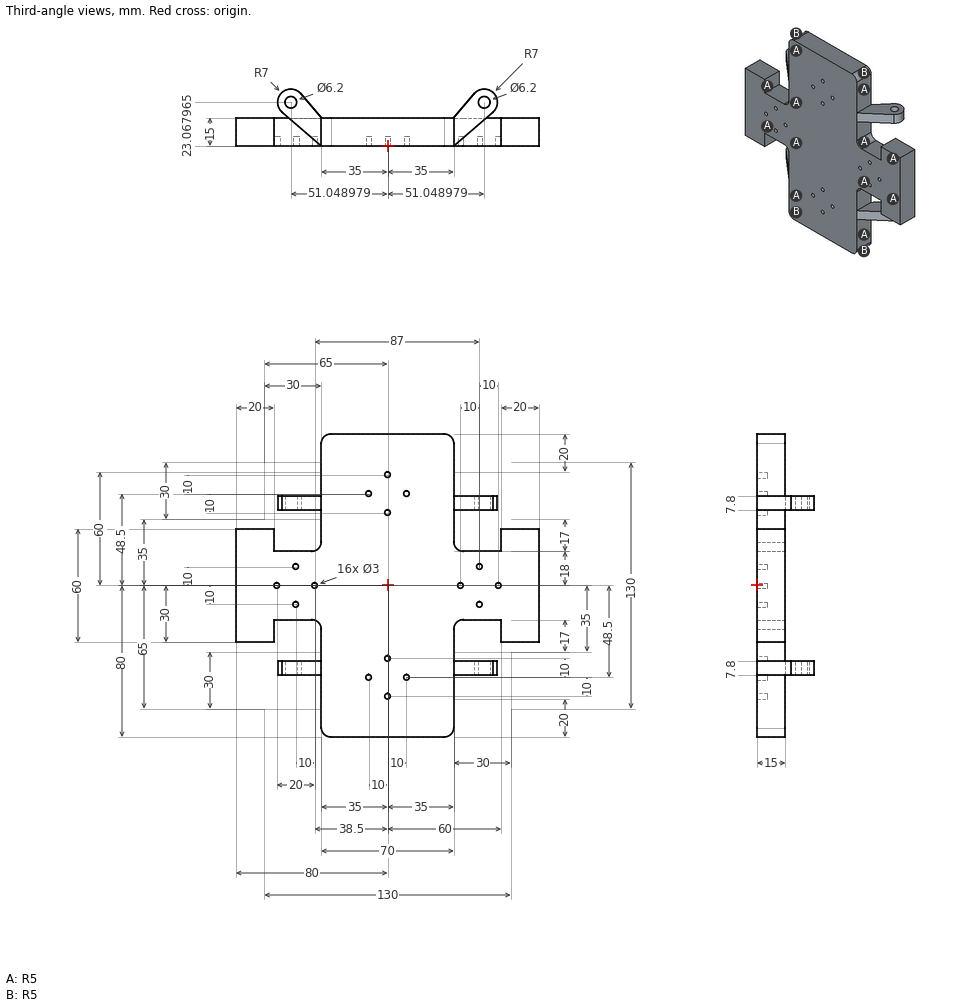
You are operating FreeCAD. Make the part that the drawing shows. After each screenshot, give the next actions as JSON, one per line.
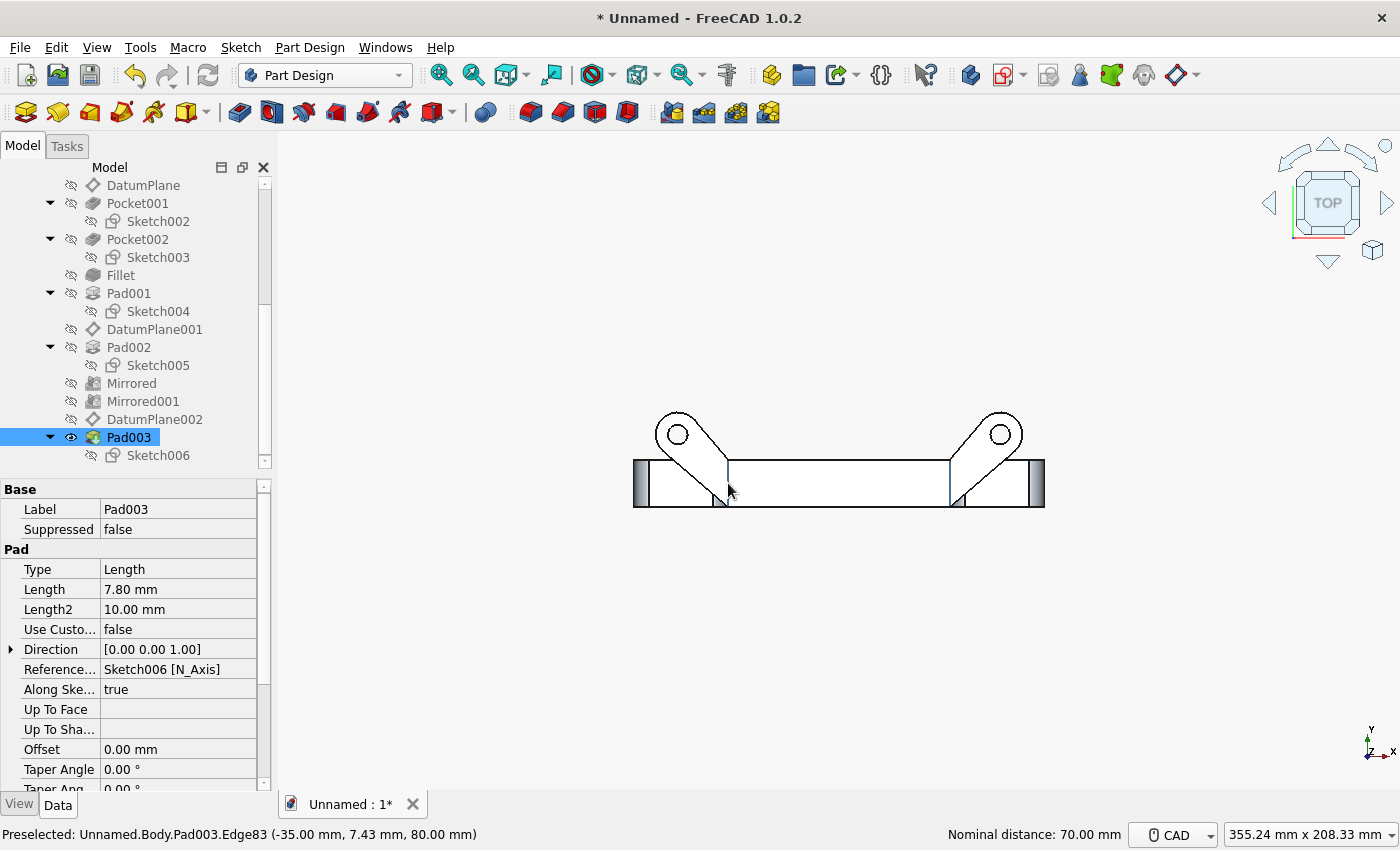
{"action": "key", "text": "1"}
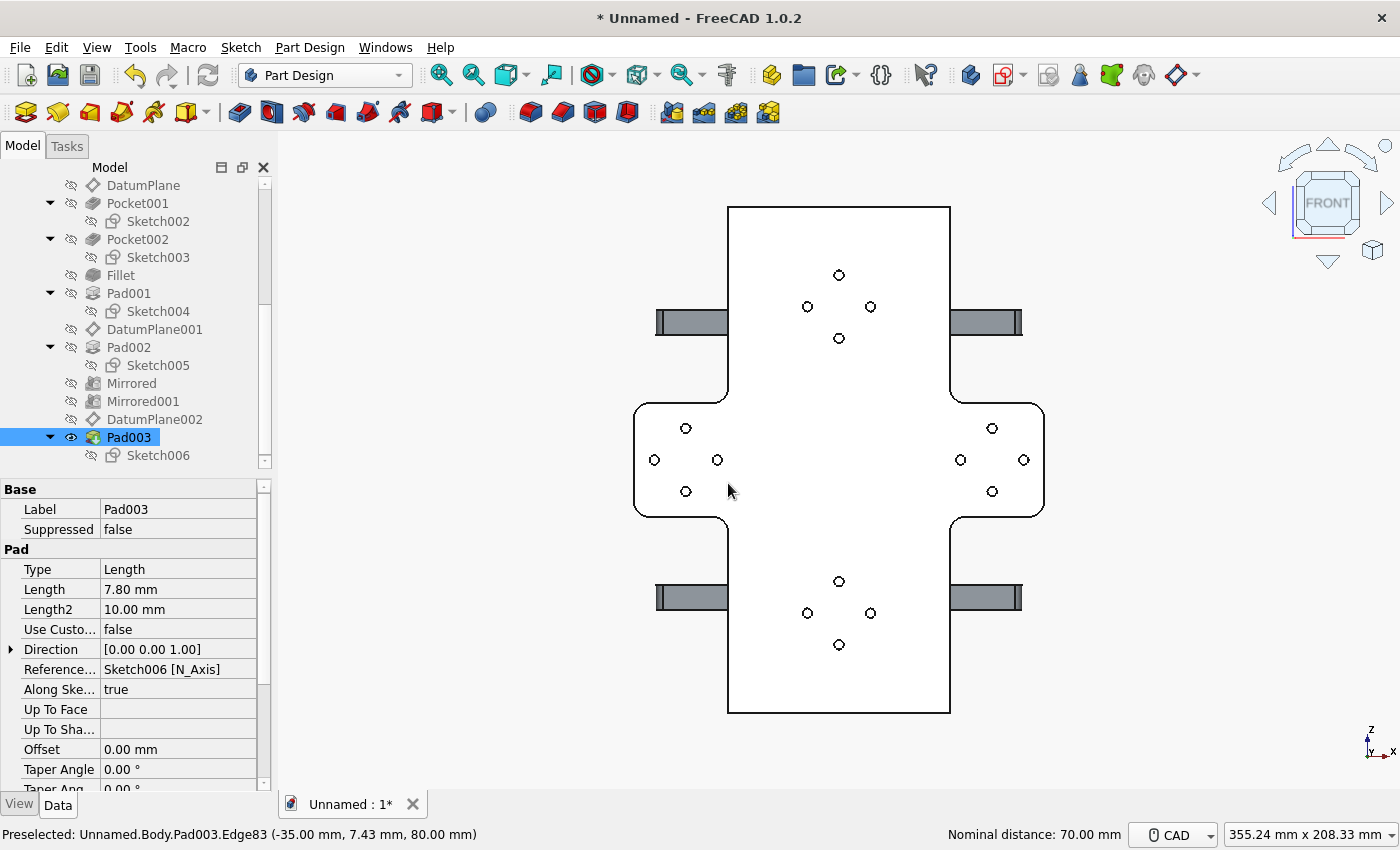
{"action": "key", "text": "3"}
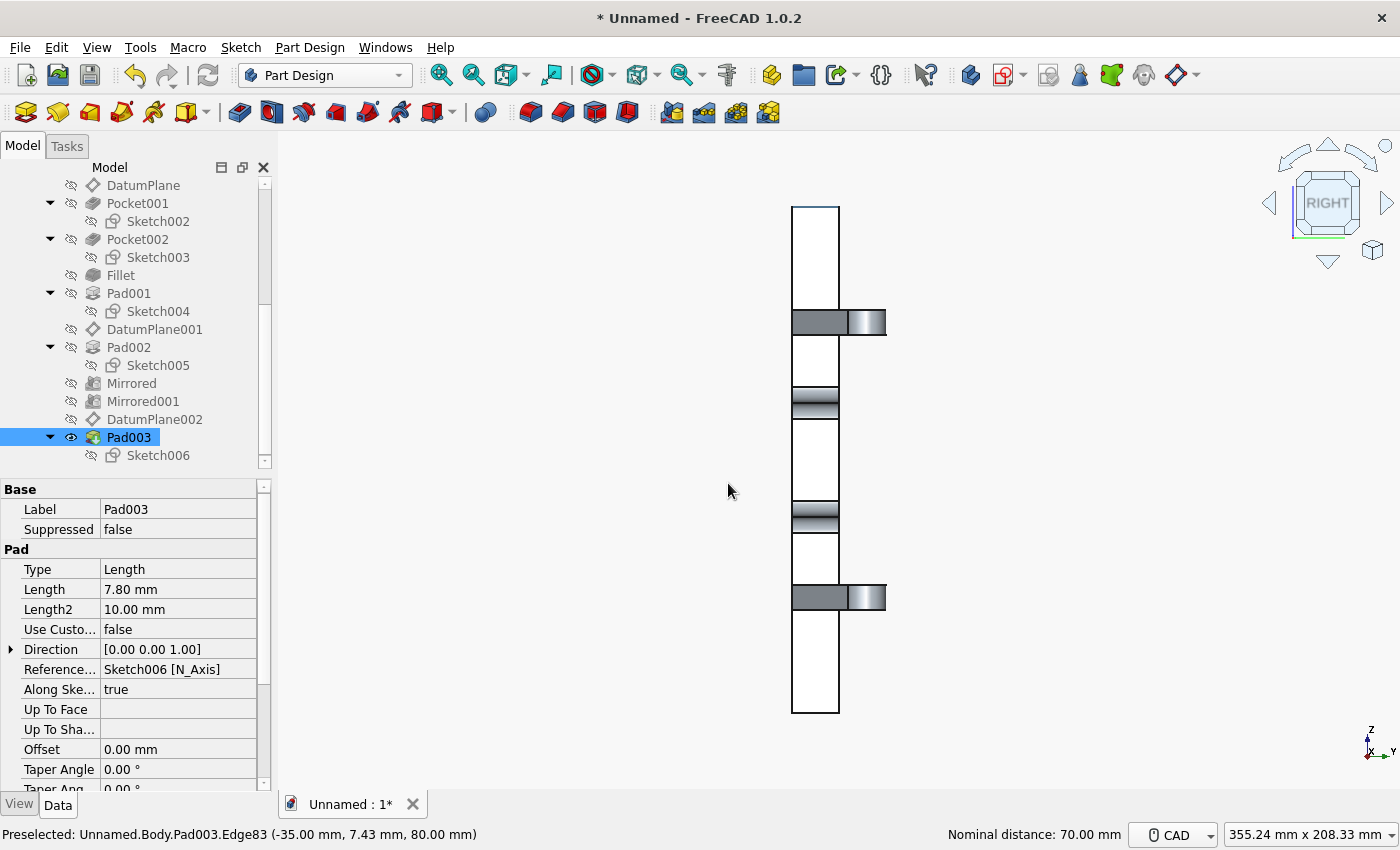
{"action": "left_click", "coordinate": [815, 712], "text": "ctrl"}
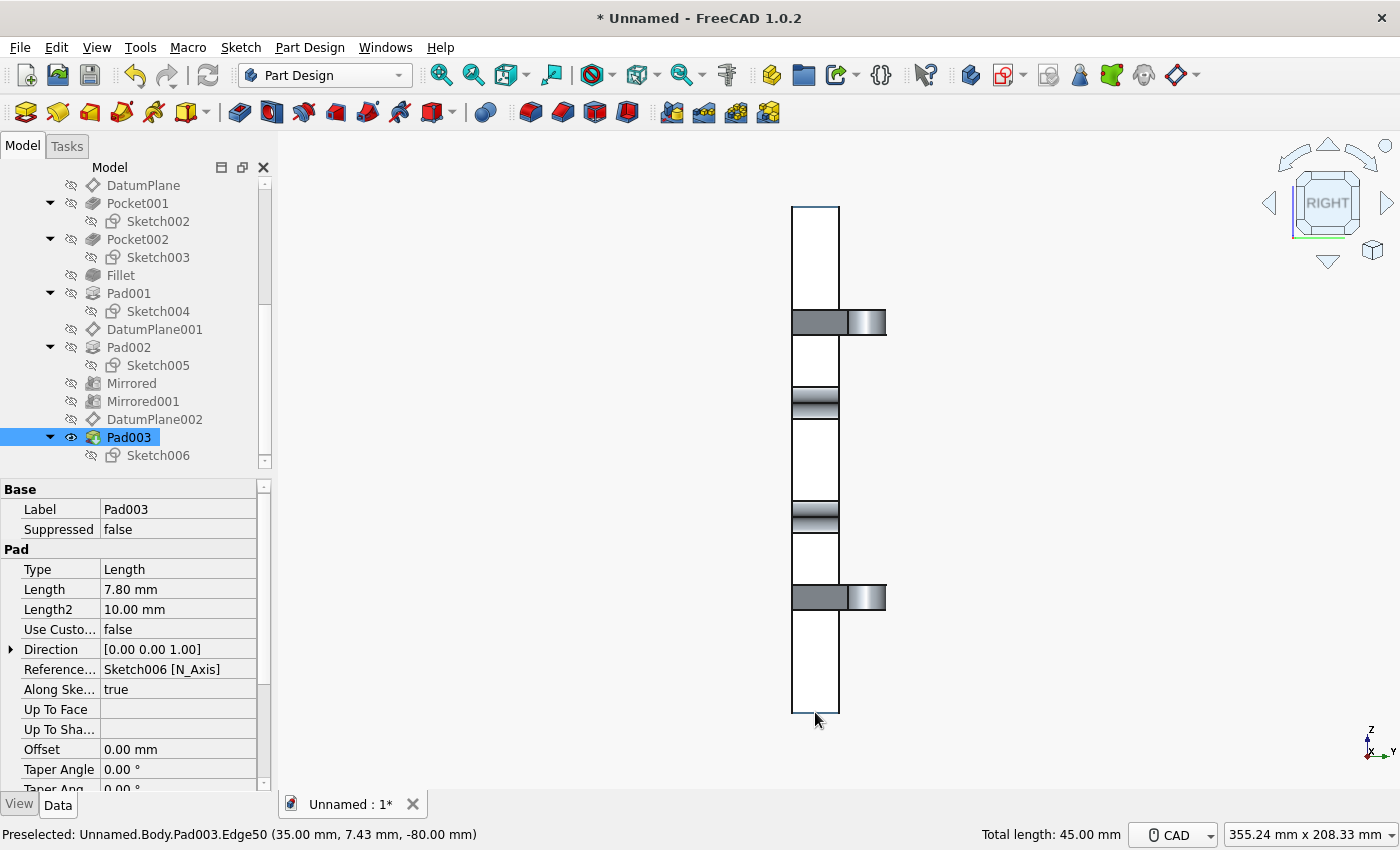
{"action": "key", "text": "5"}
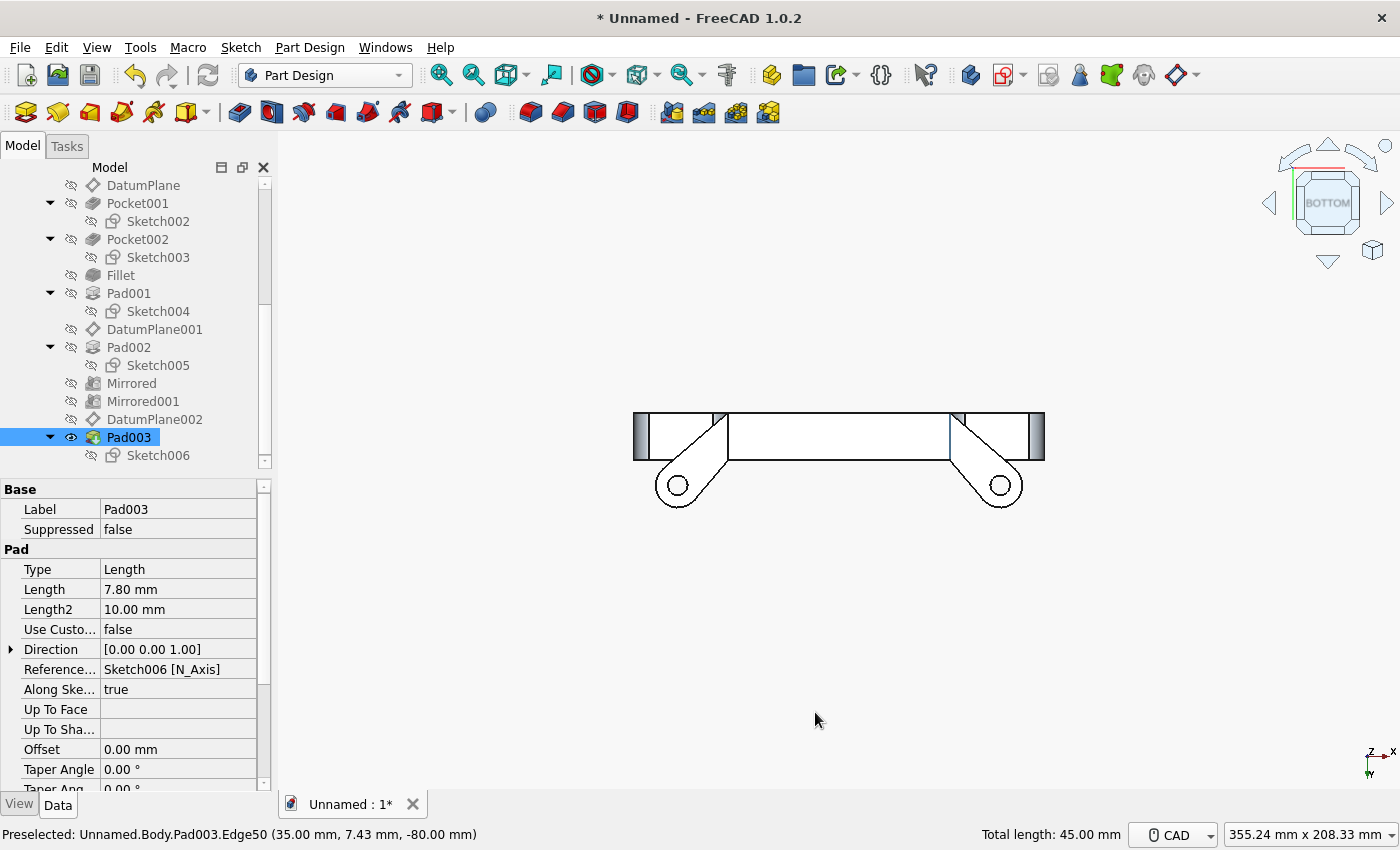
{"action": "left_click", "coordinate": [442, 76]}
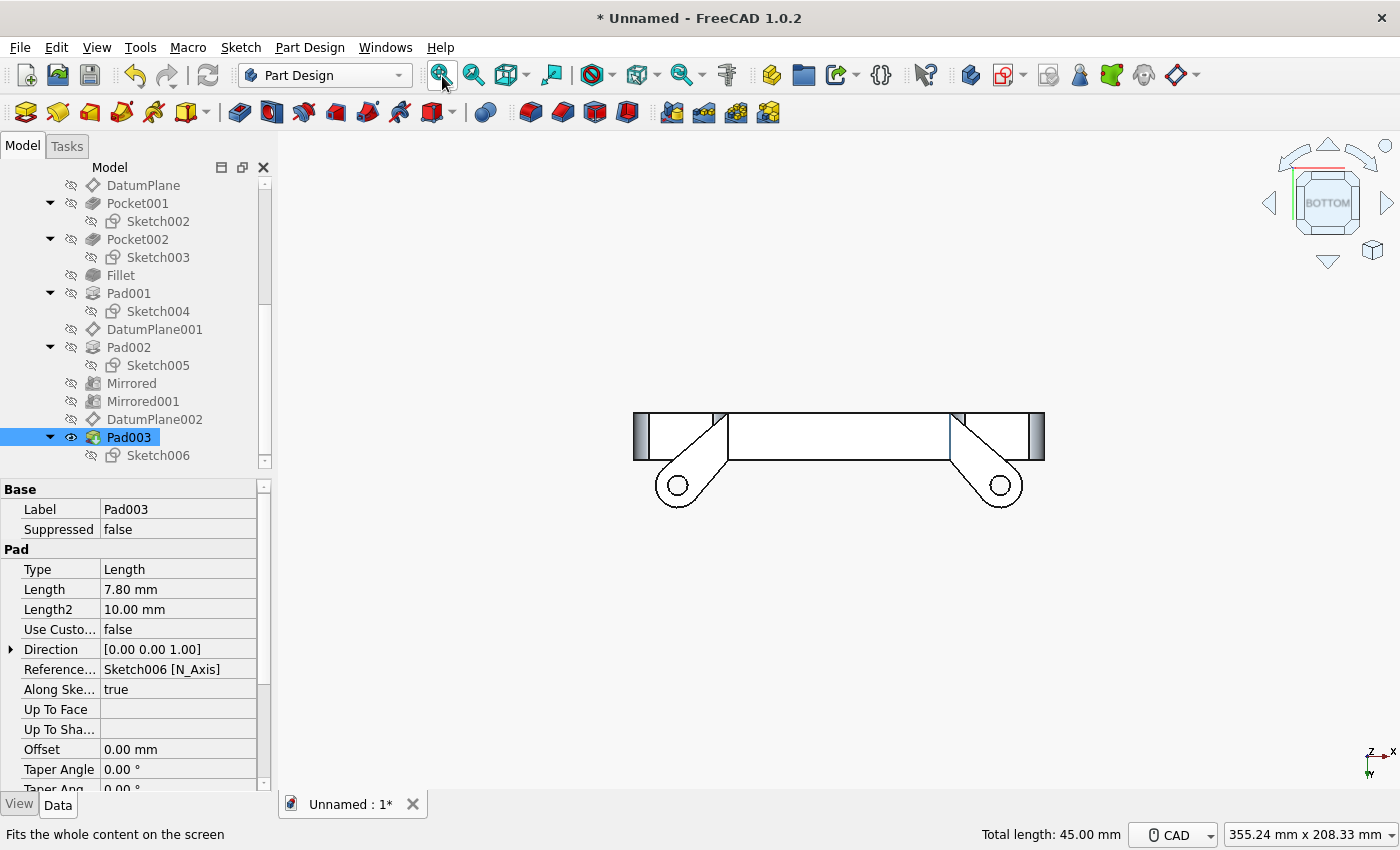
{"action": "left_click", "coordinate": [728, 435], "text": "ctrl"}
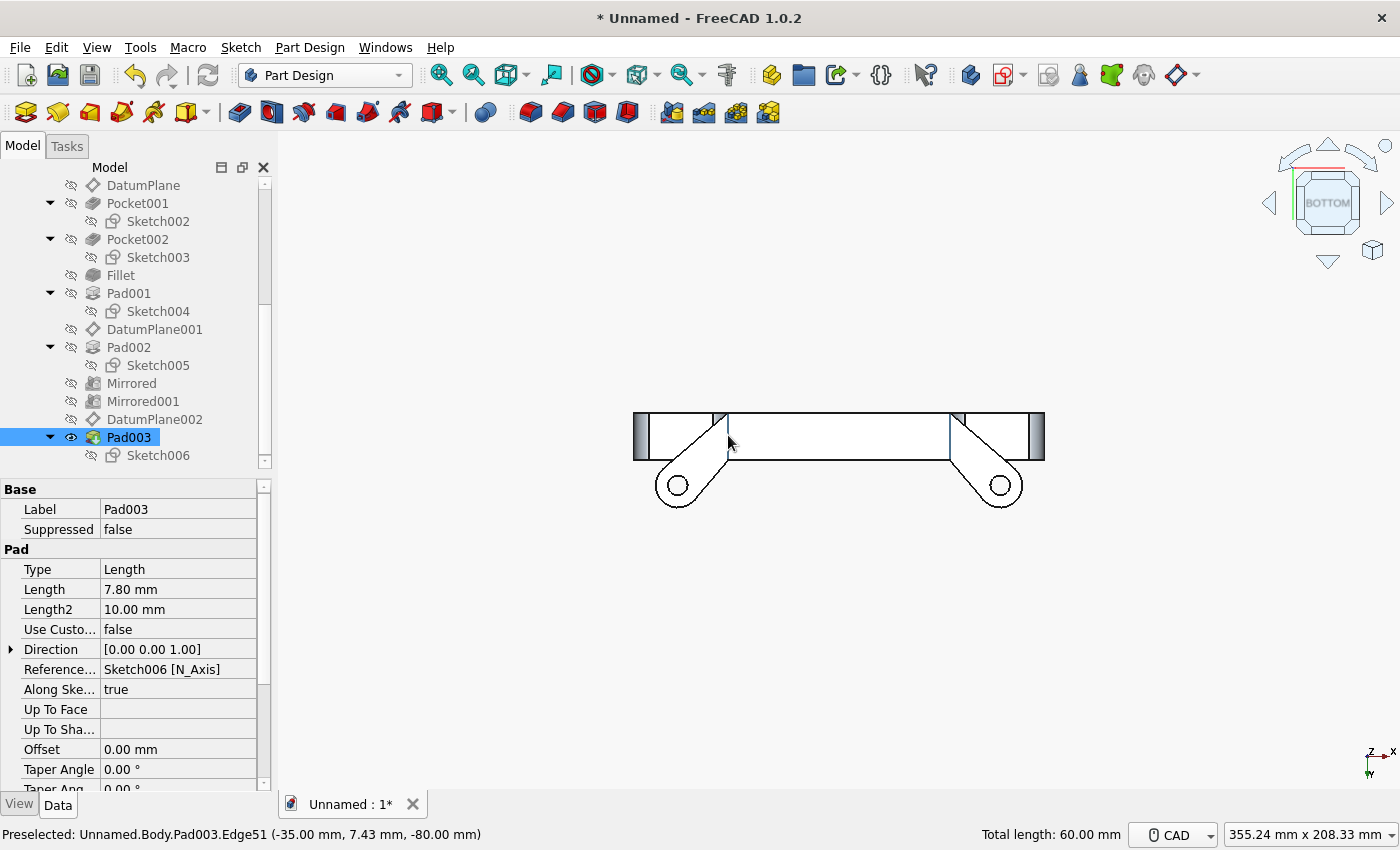
{"action": "left_click", "coordinate": [532, 112]}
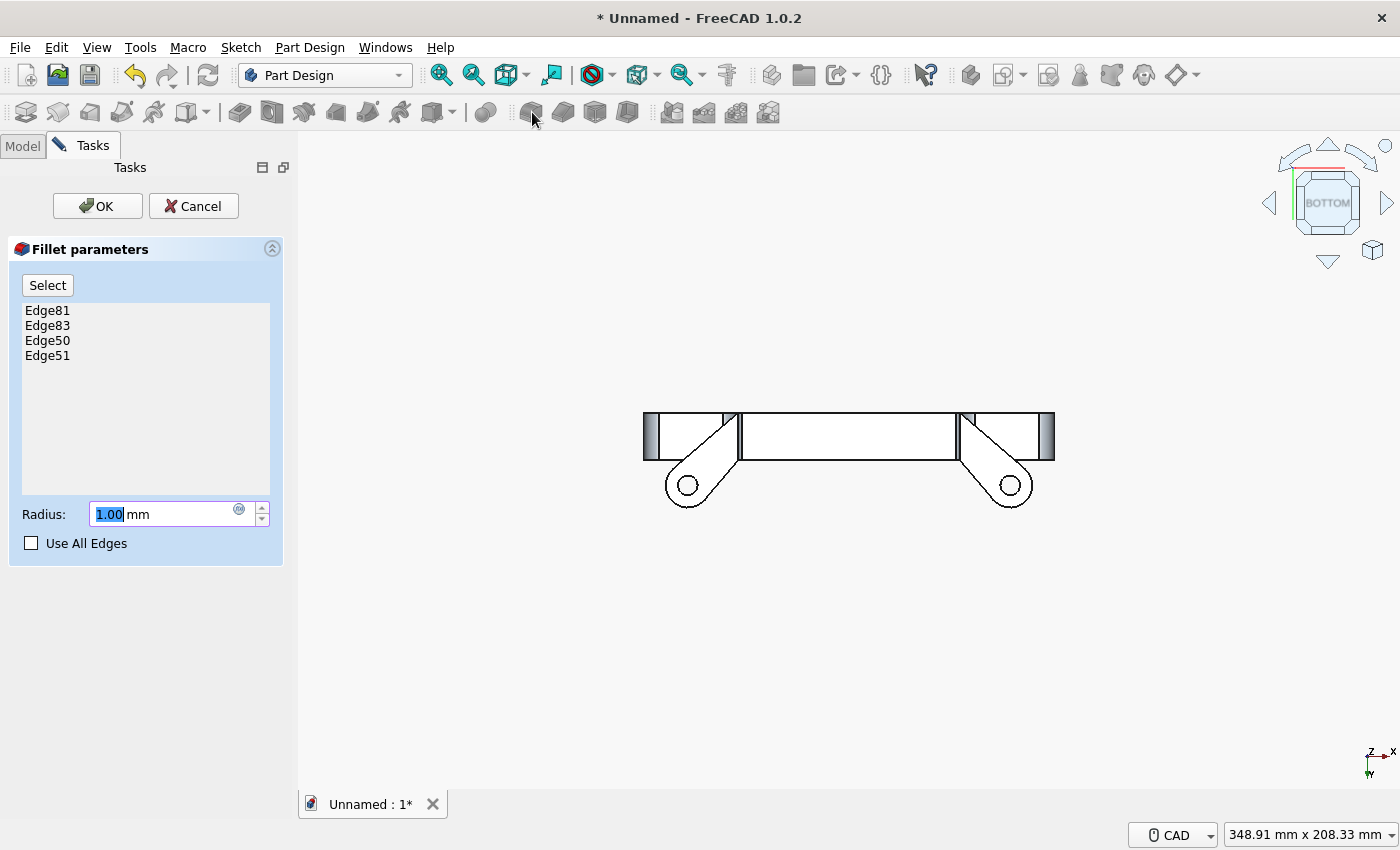
{"action": "type", "text": "5"}
{"action": "key", "text": "Tab"}